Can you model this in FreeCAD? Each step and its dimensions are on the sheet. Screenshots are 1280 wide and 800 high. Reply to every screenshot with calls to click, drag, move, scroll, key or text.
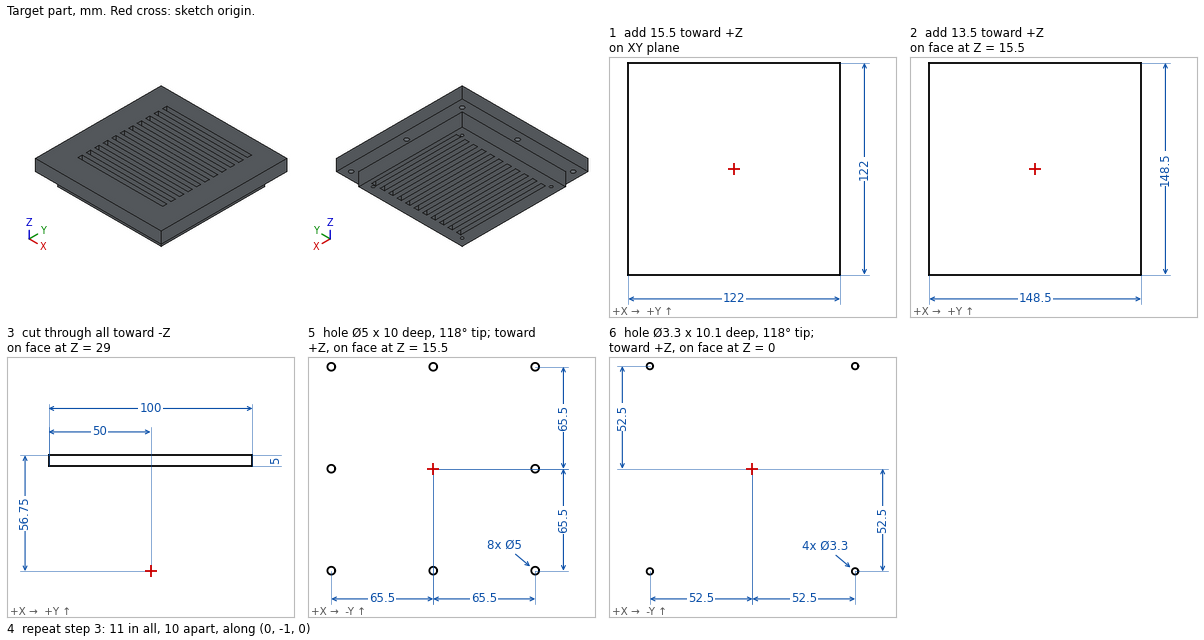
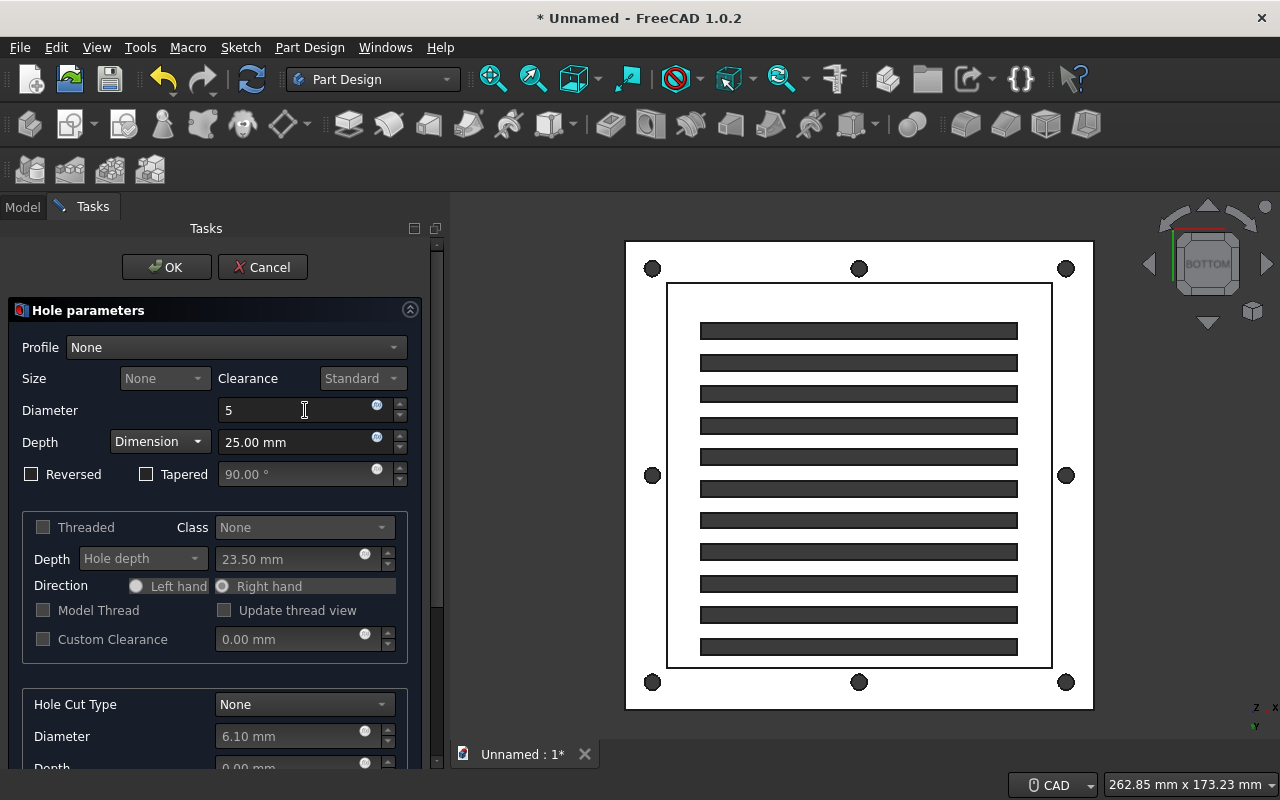
triple_click(305, 442)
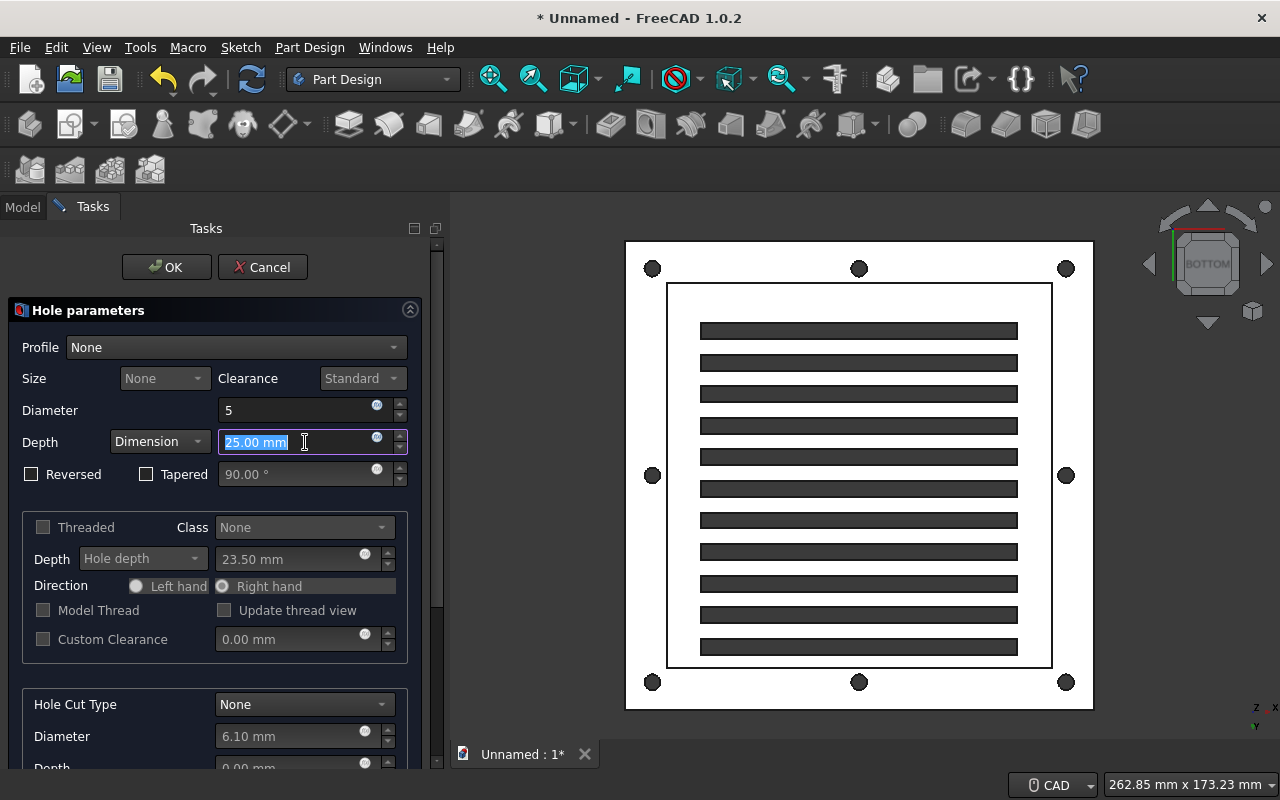
text(10)
key(Tab)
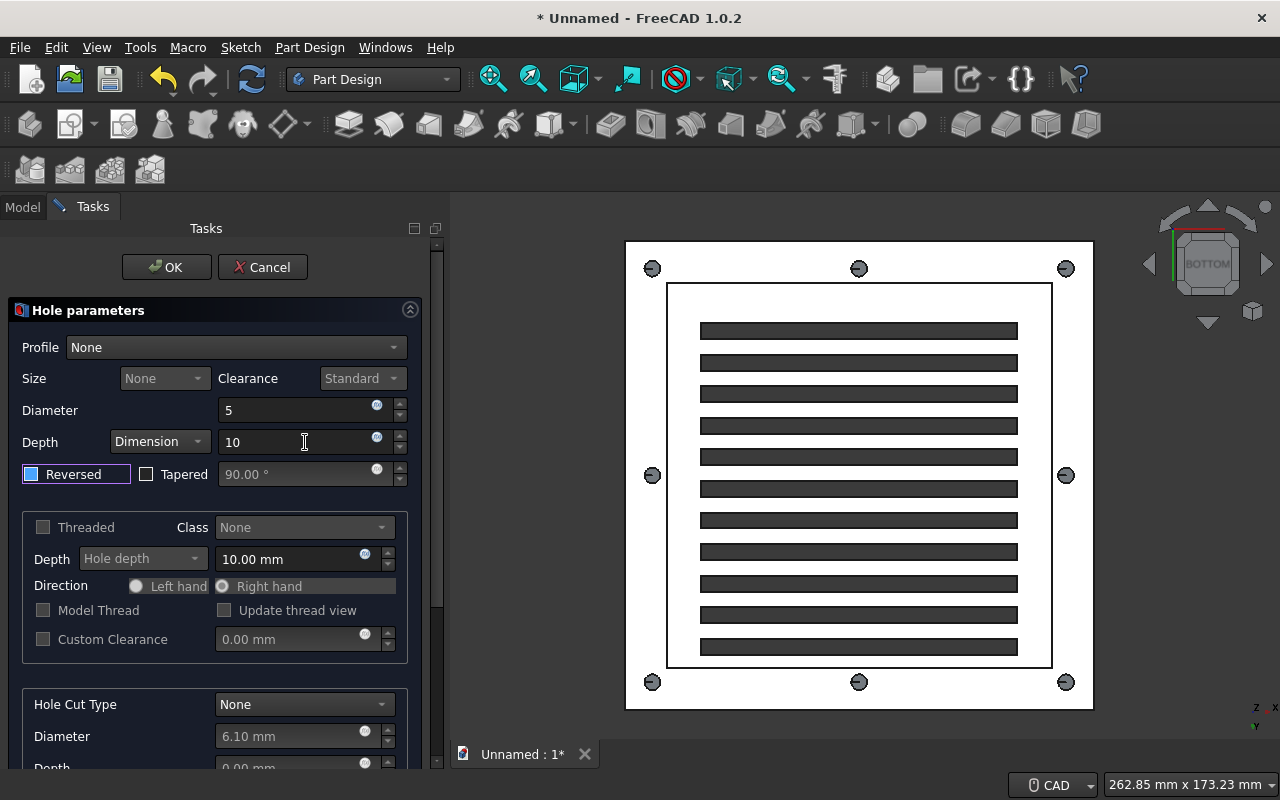
click(167, 267)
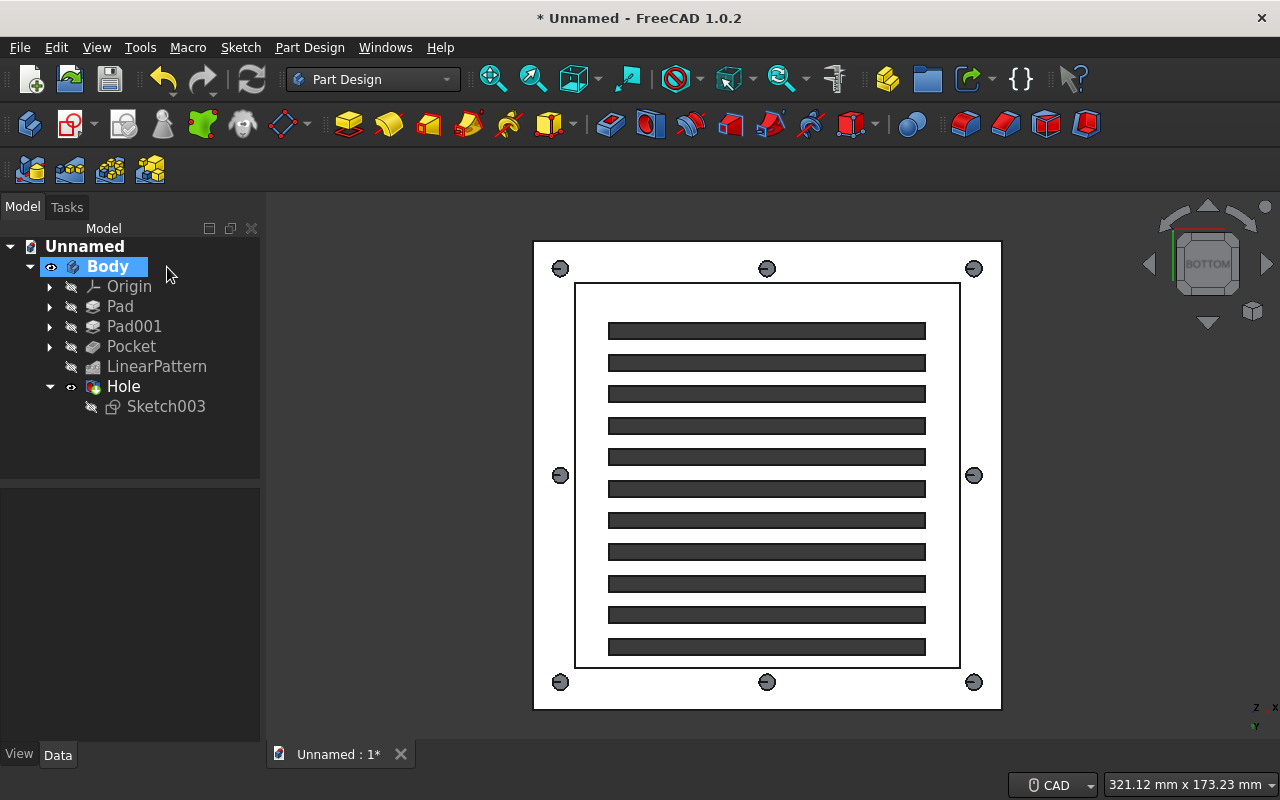
click(932, 309)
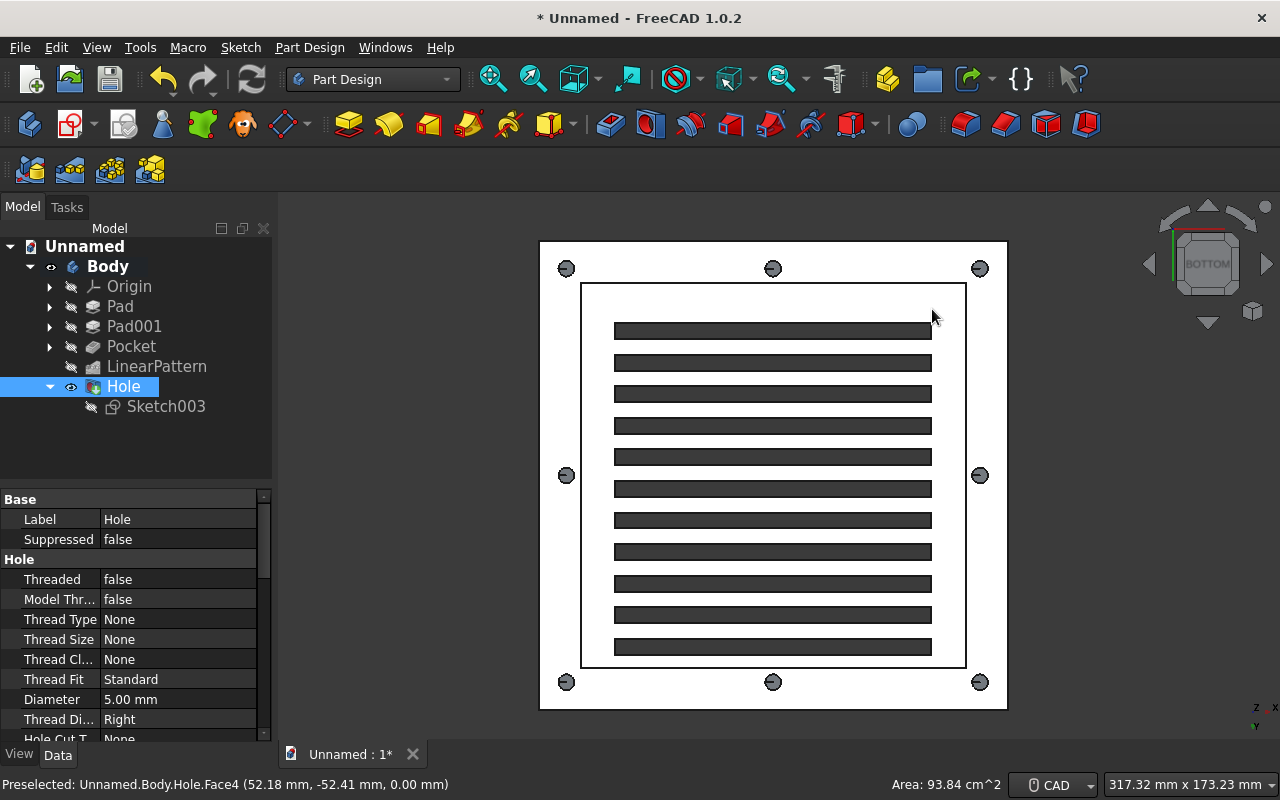
click(70, 124)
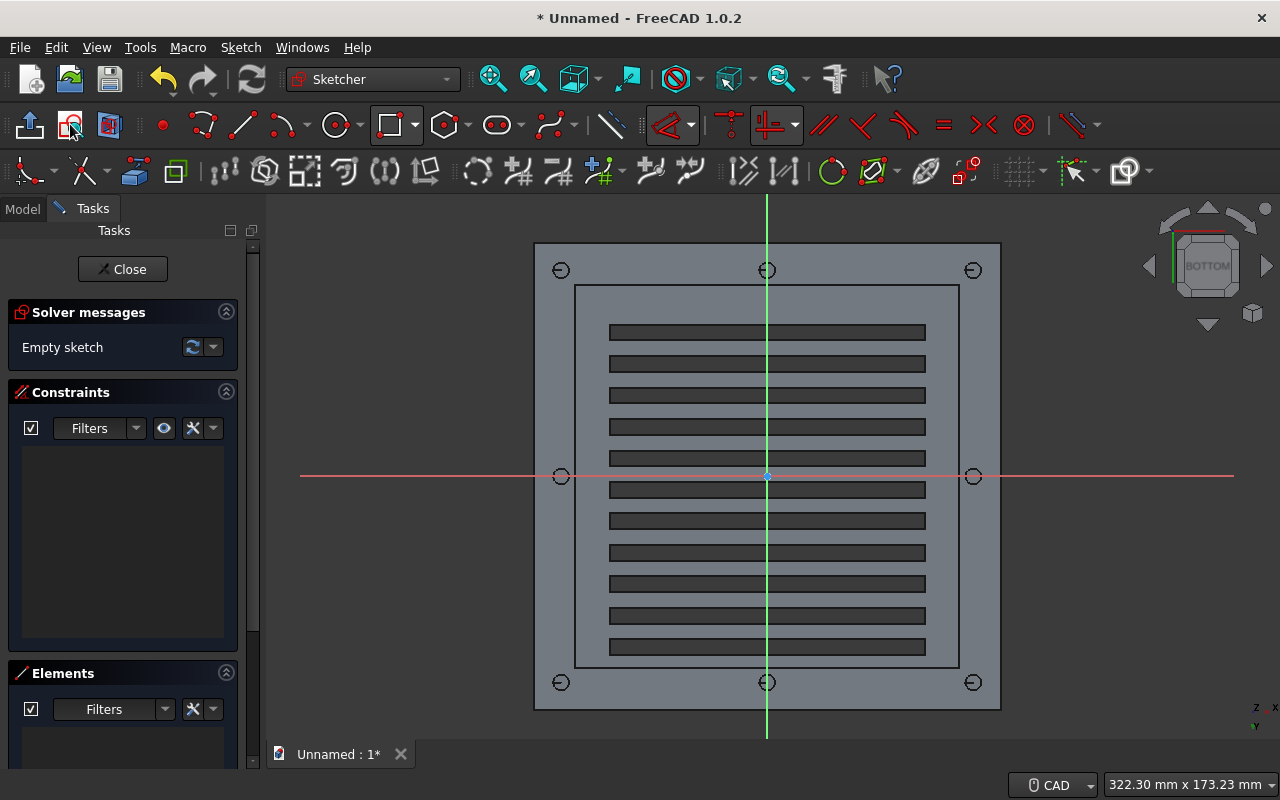
click(336, 126)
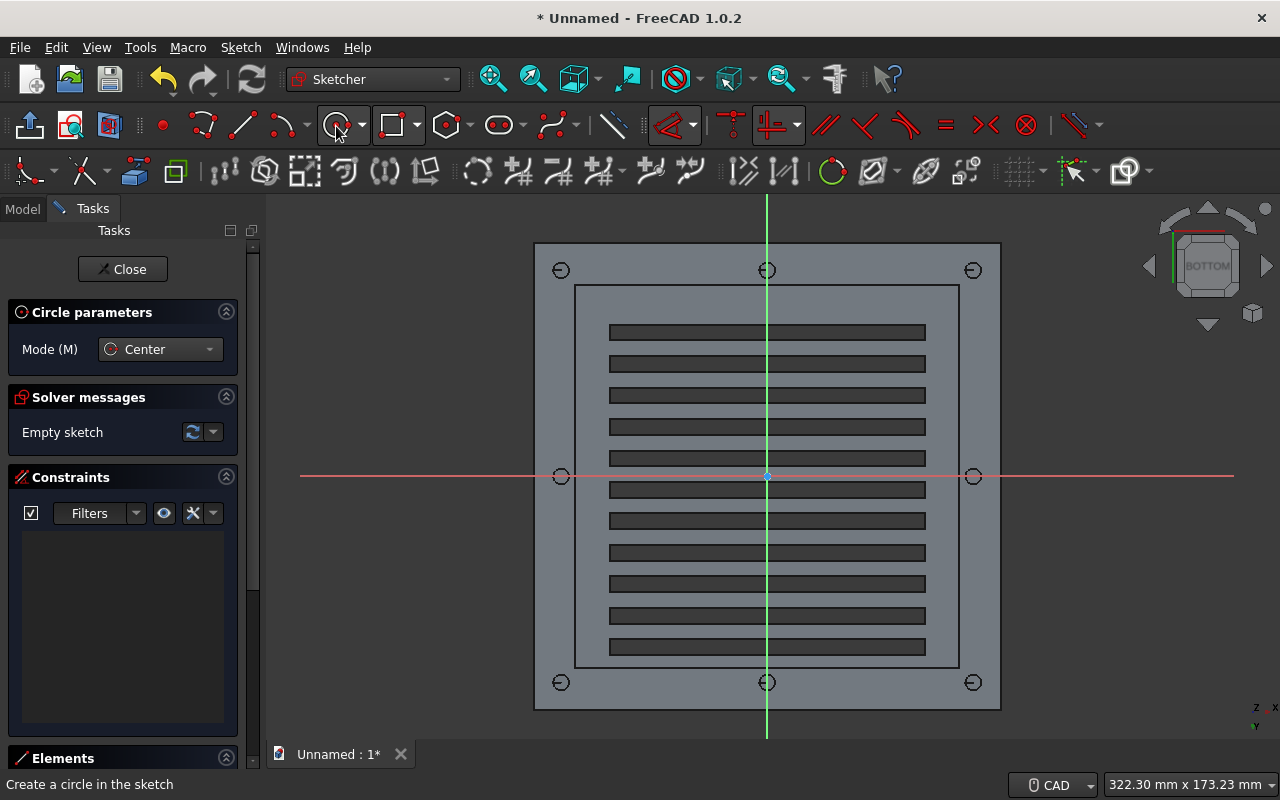
scroll(932, 642, up, 8)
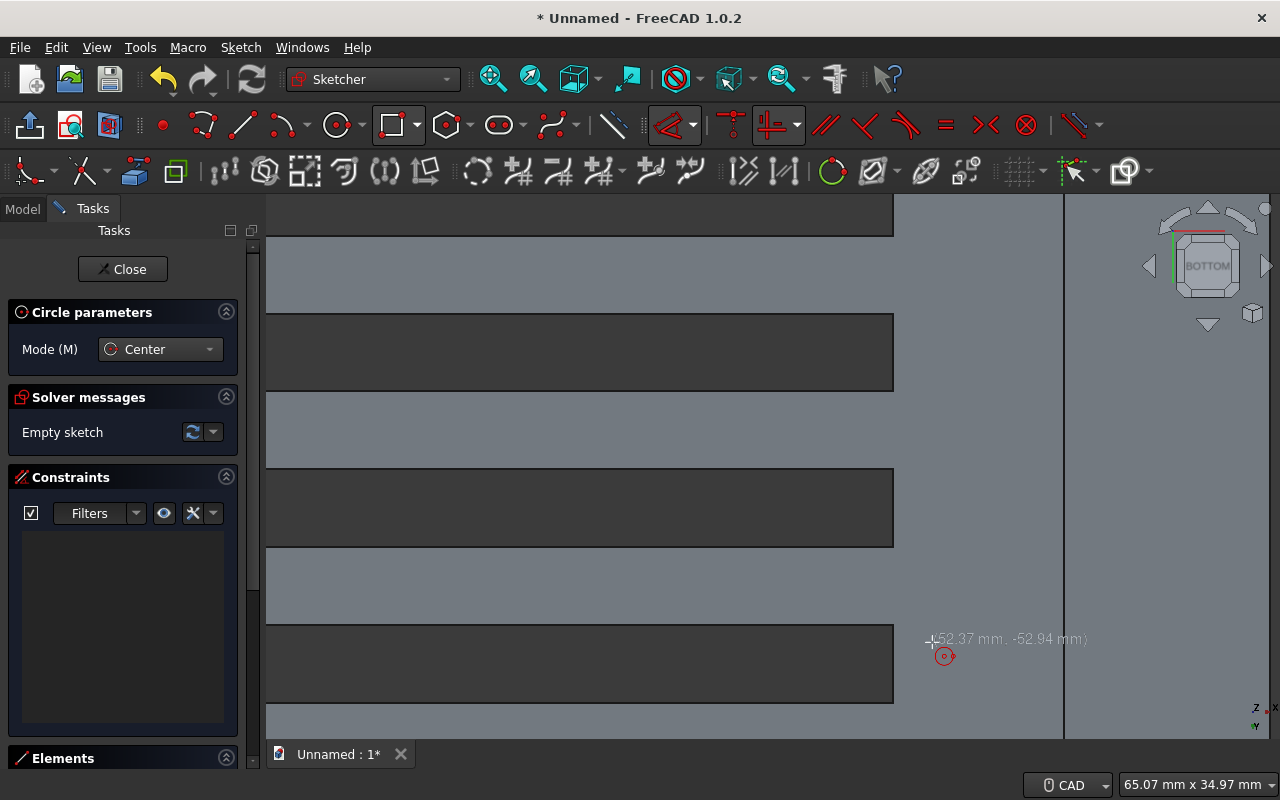
scroll(854, 630, down, 8)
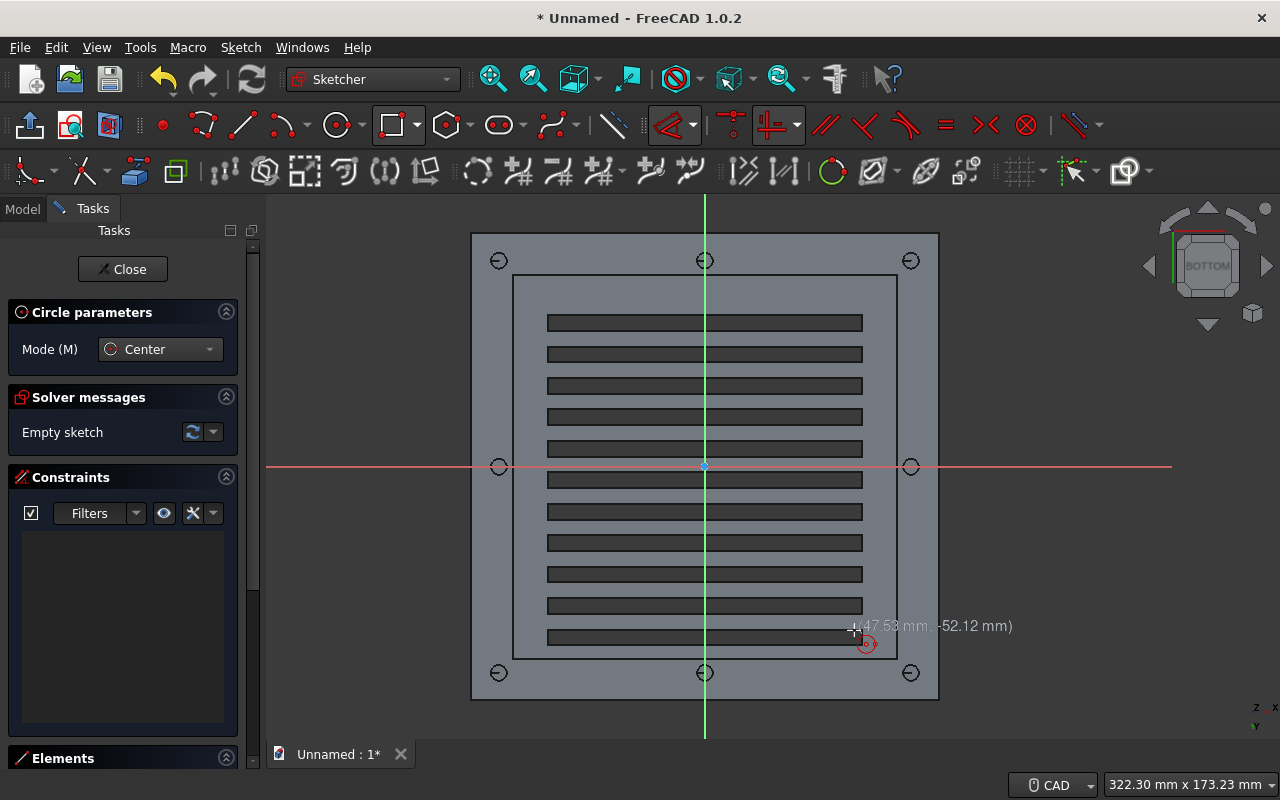
click(870, 632)
move(874, 628)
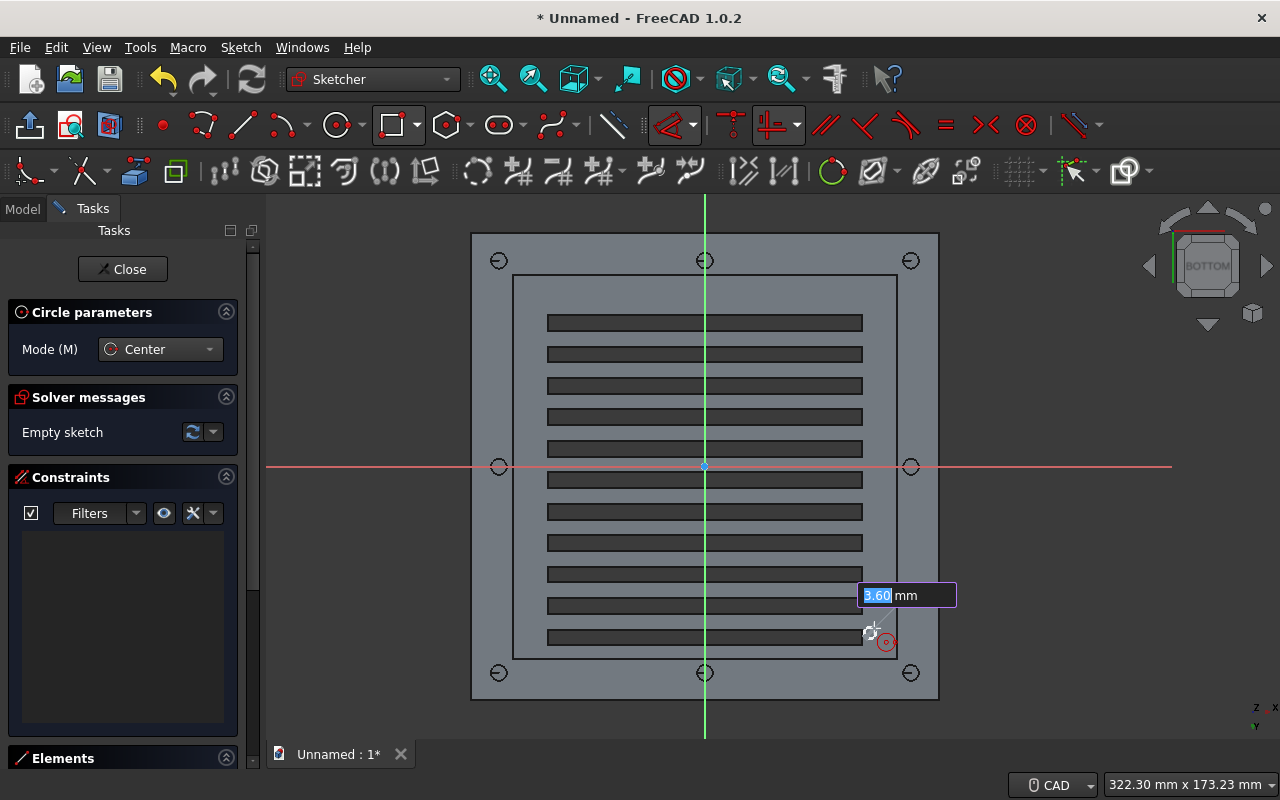
text(3.3)
key(Return)